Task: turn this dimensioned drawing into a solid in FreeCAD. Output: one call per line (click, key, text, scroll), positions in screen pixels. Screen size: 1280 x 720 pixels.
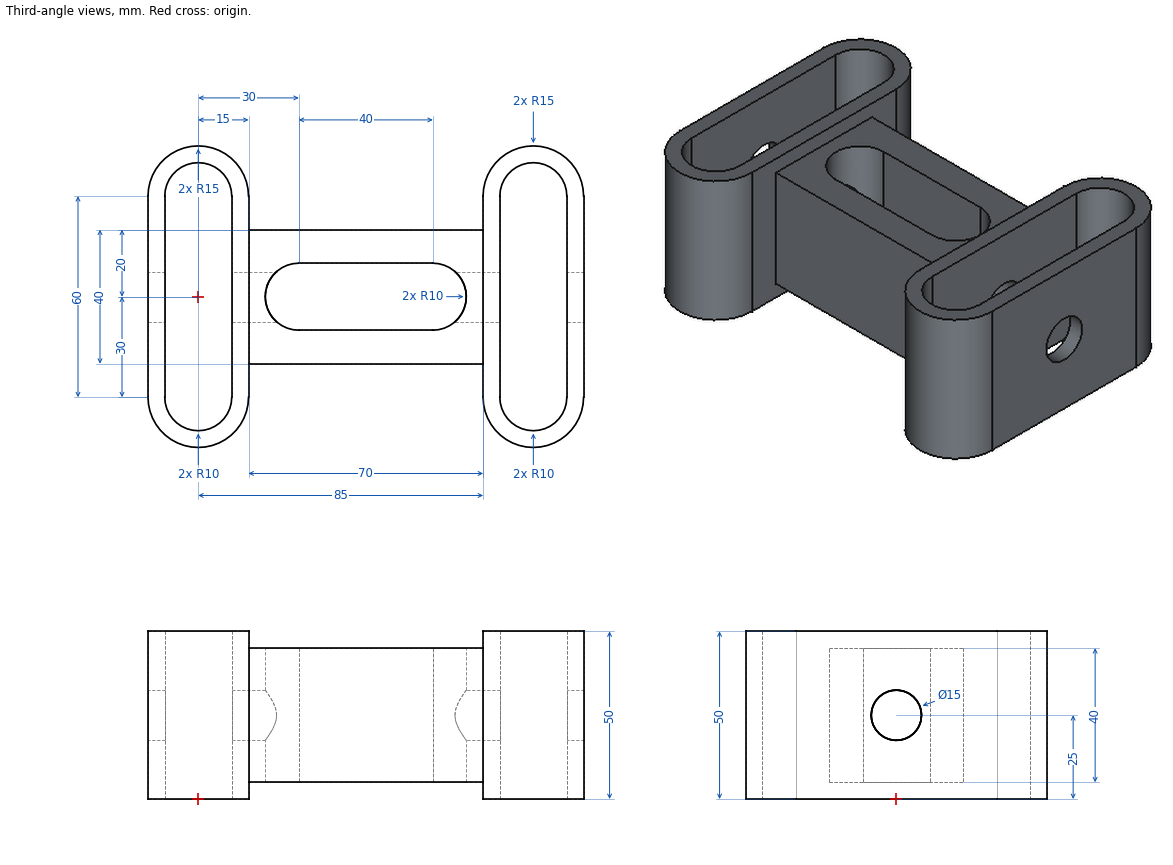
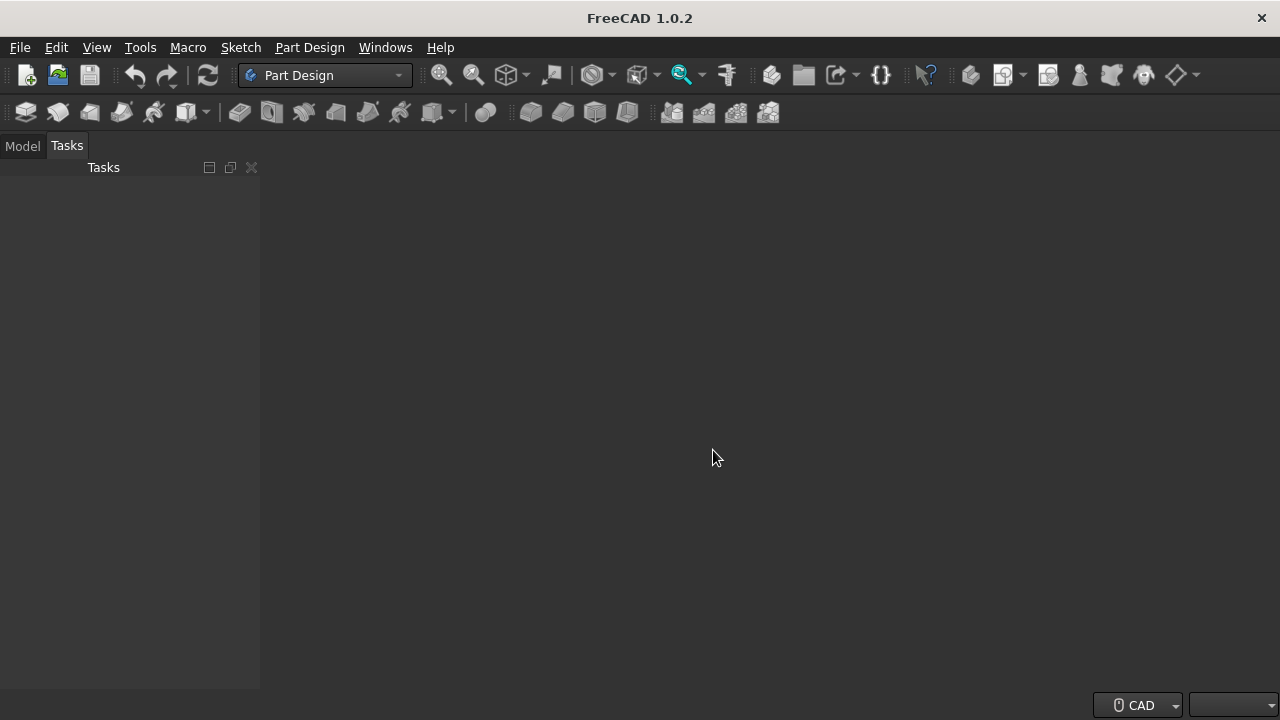
click(26, 76)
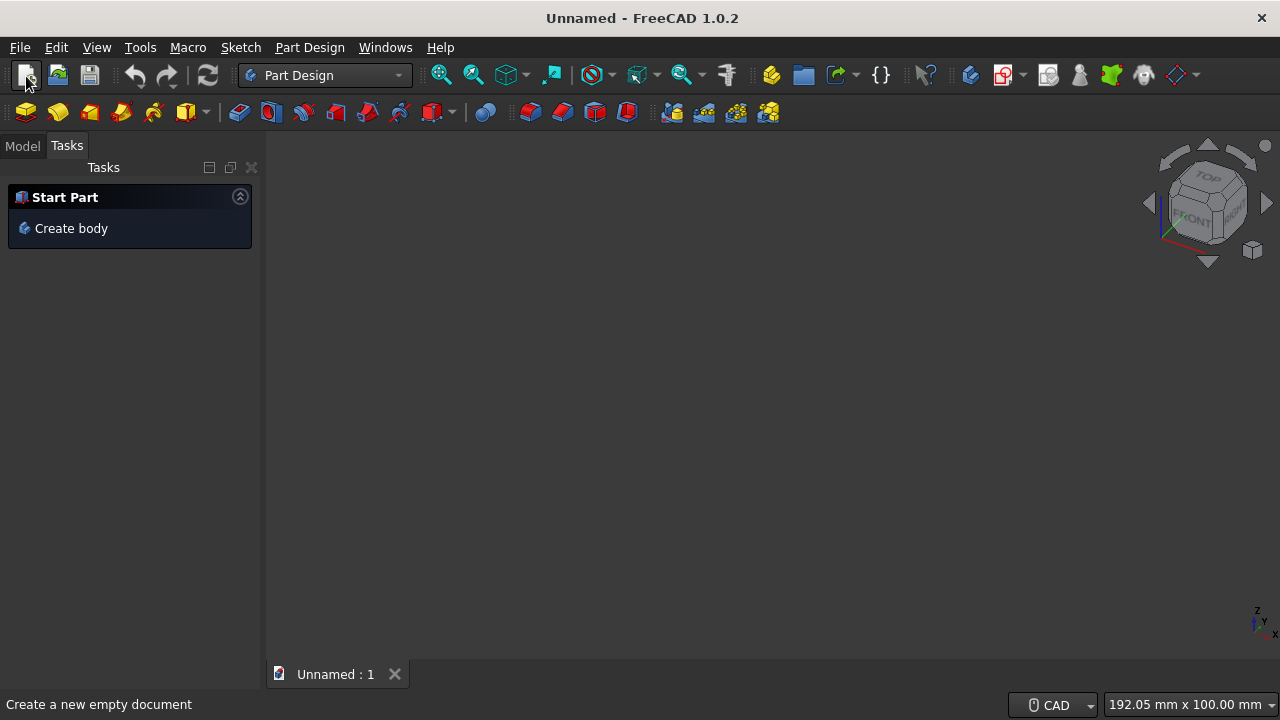
click(1004, 76)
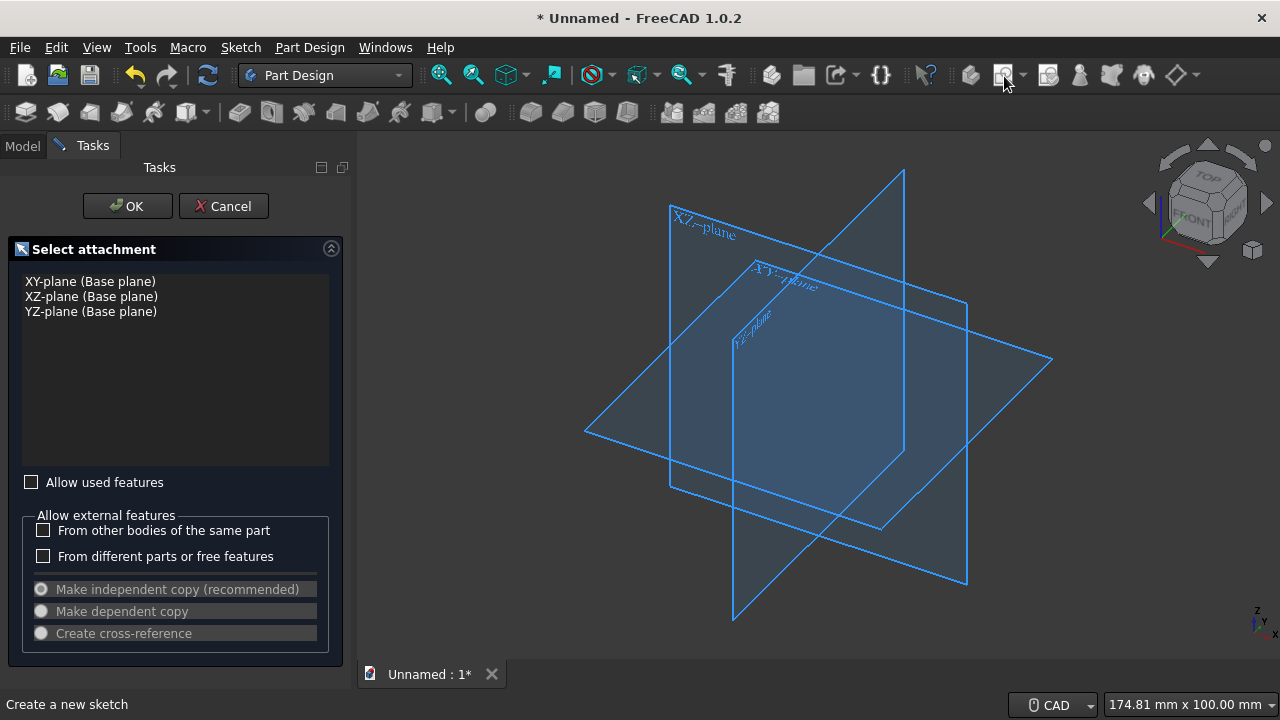
click(82, 282)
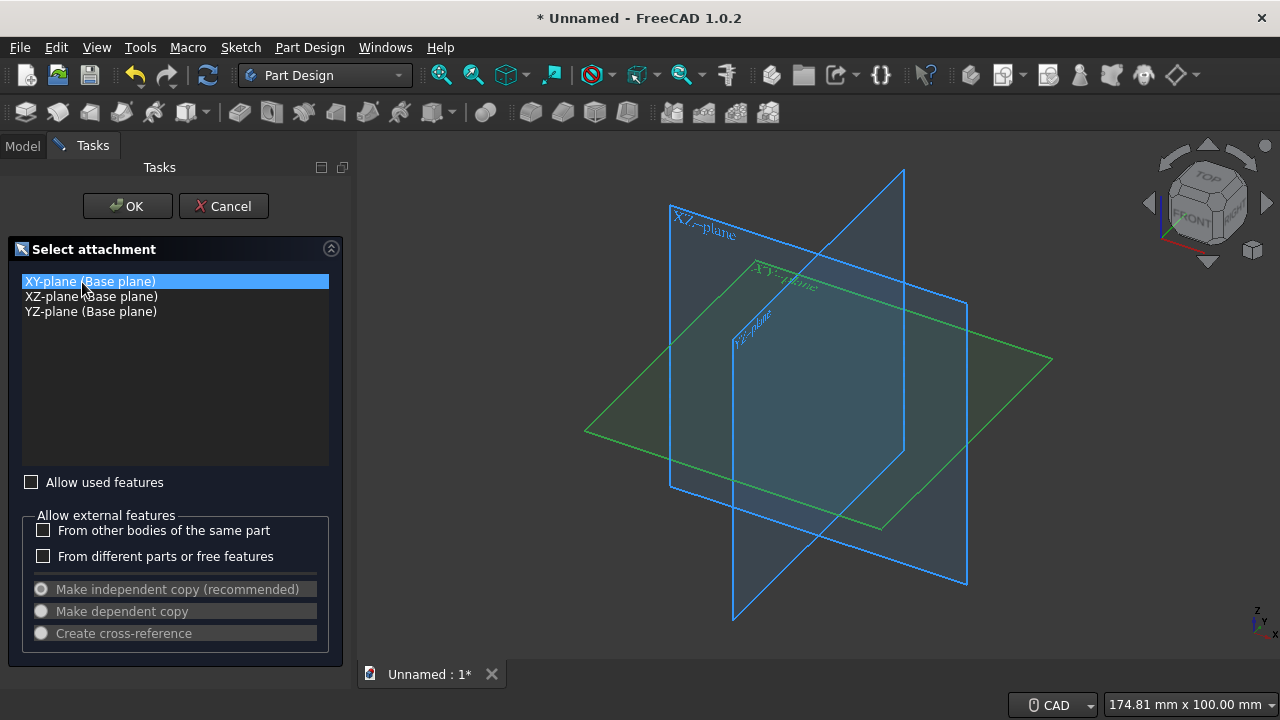
click(128, 206)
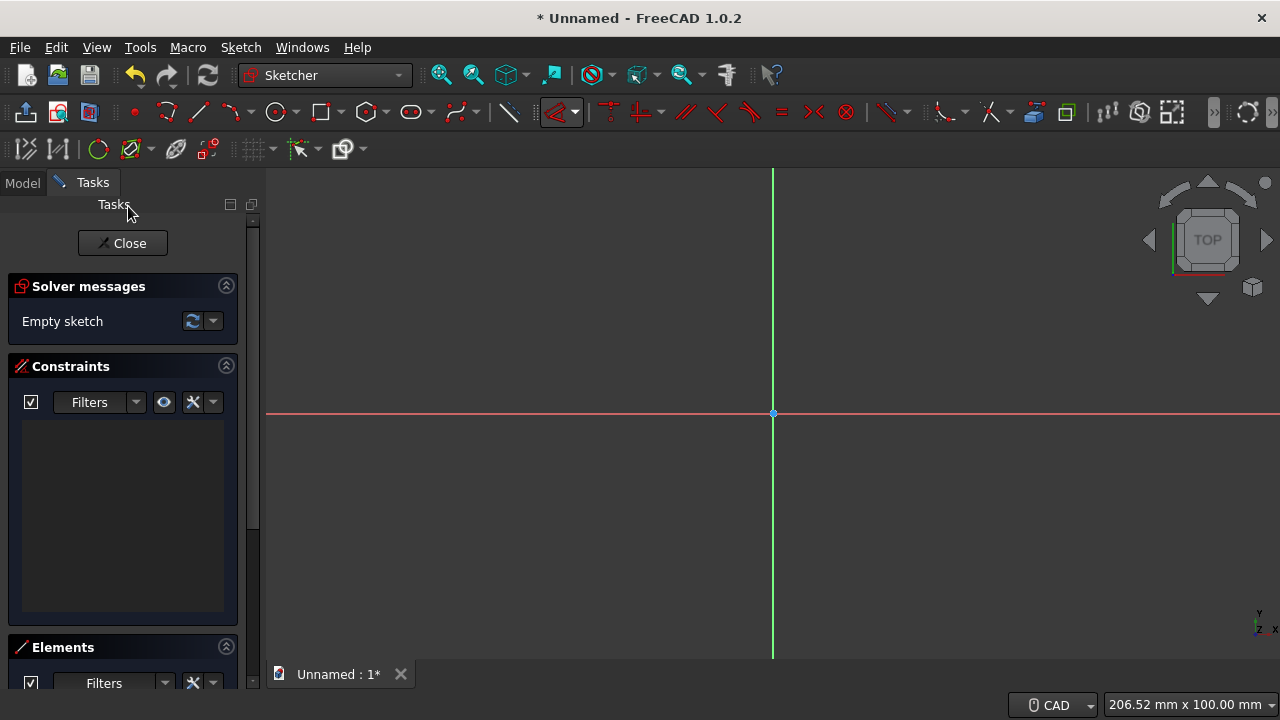
scroll(565, 414, down, 2)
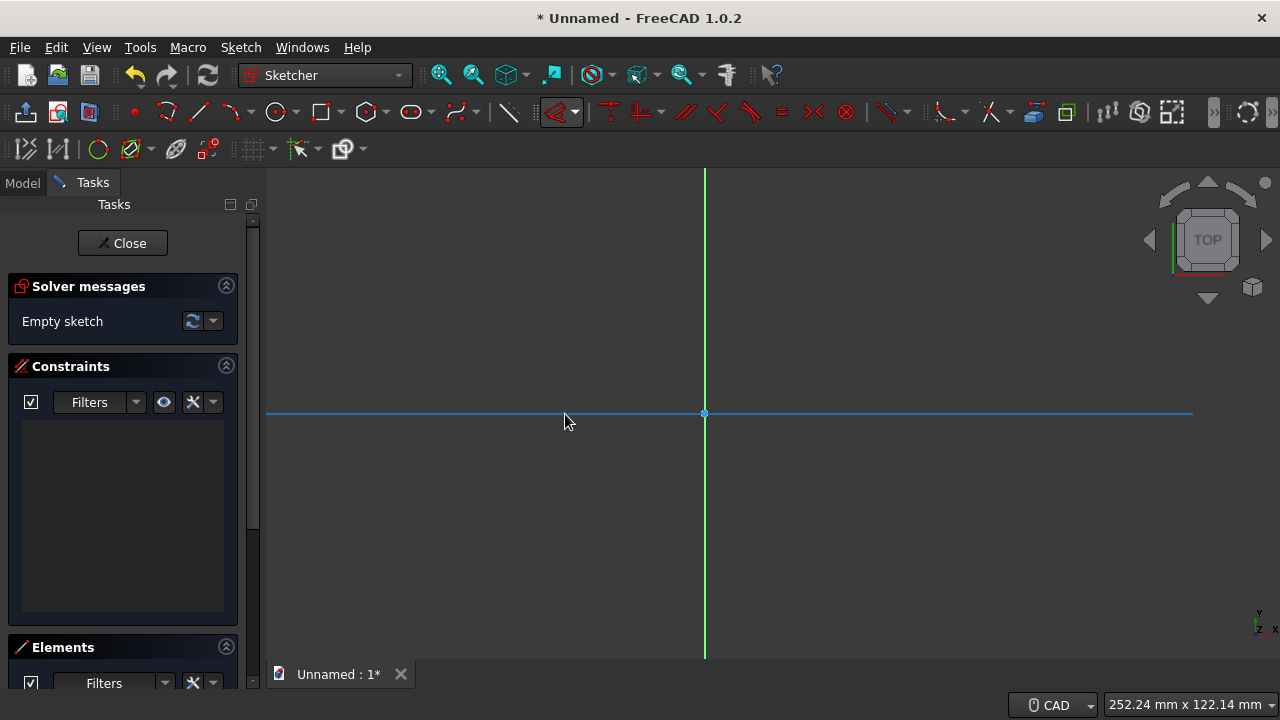
click(412, 112)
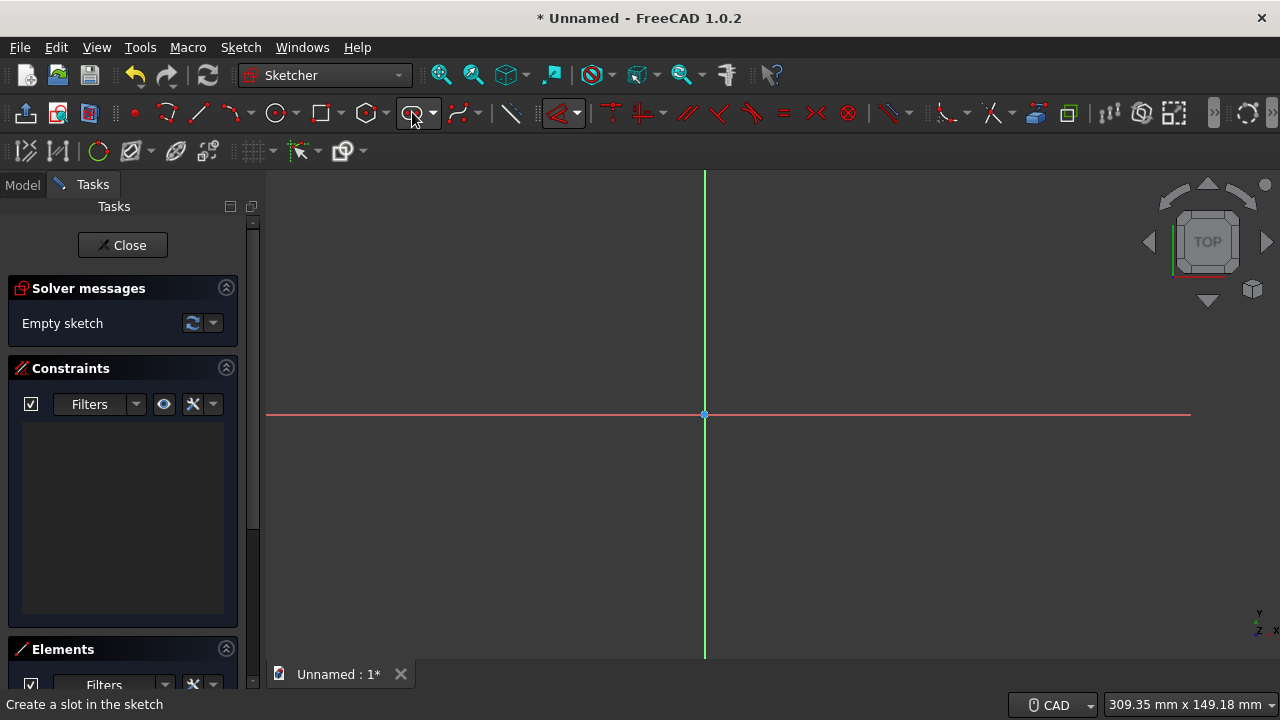
click(705, 513)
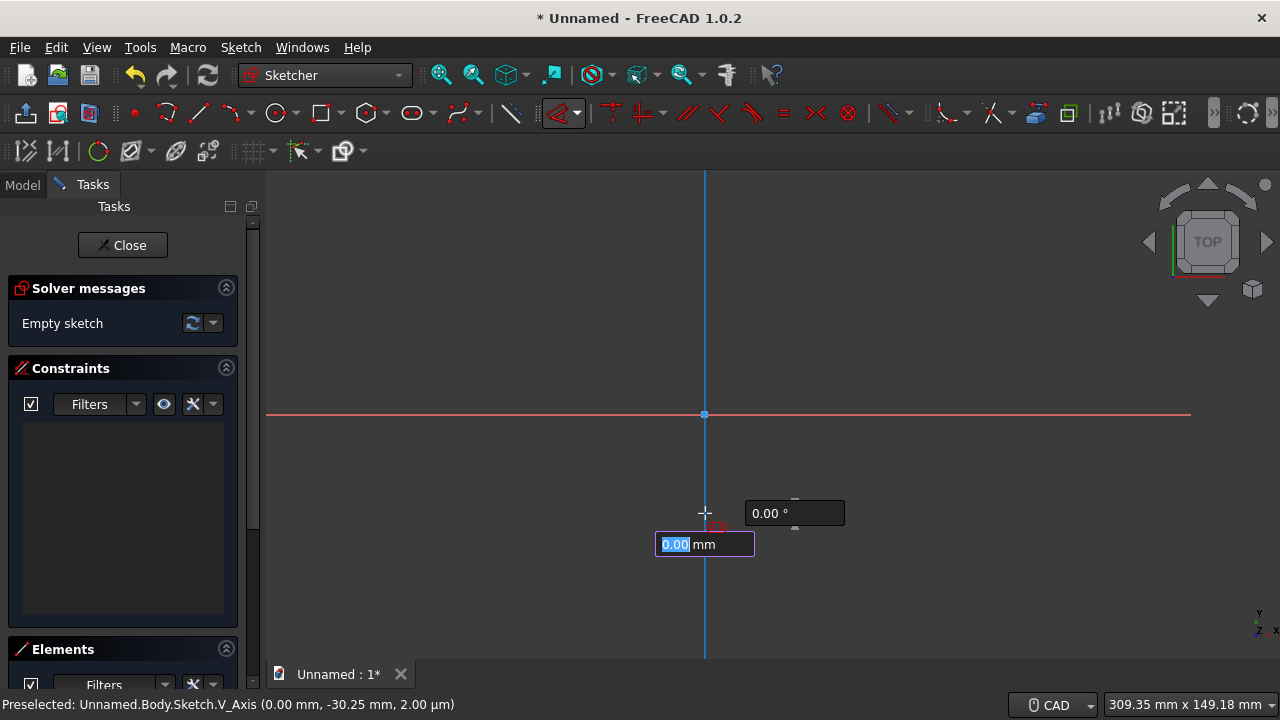
click(714, 316)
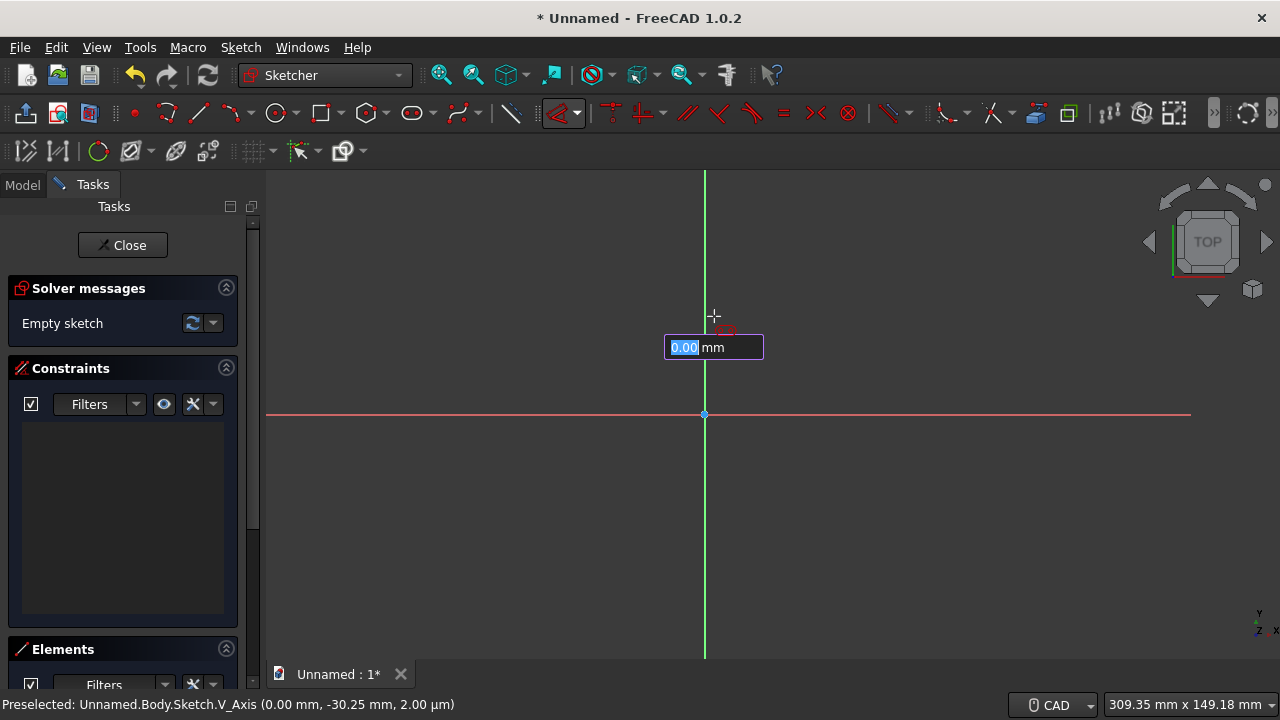
click(754, 444)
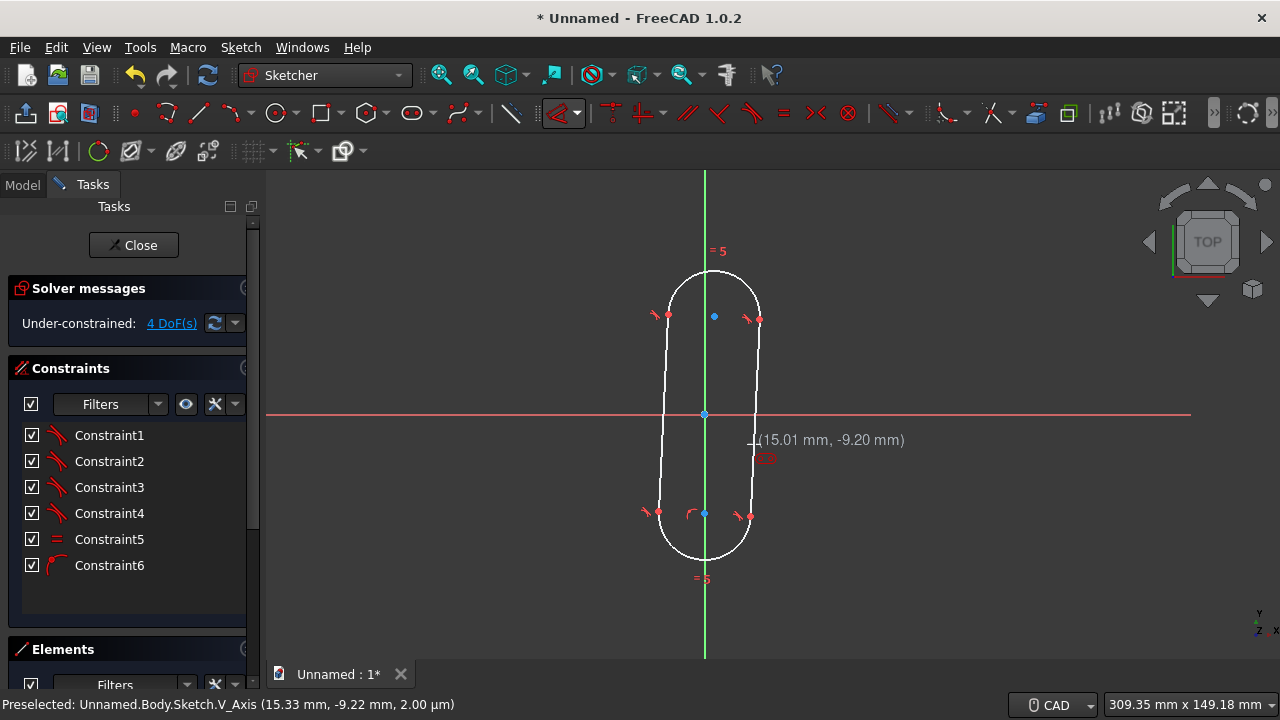
click(705, 514)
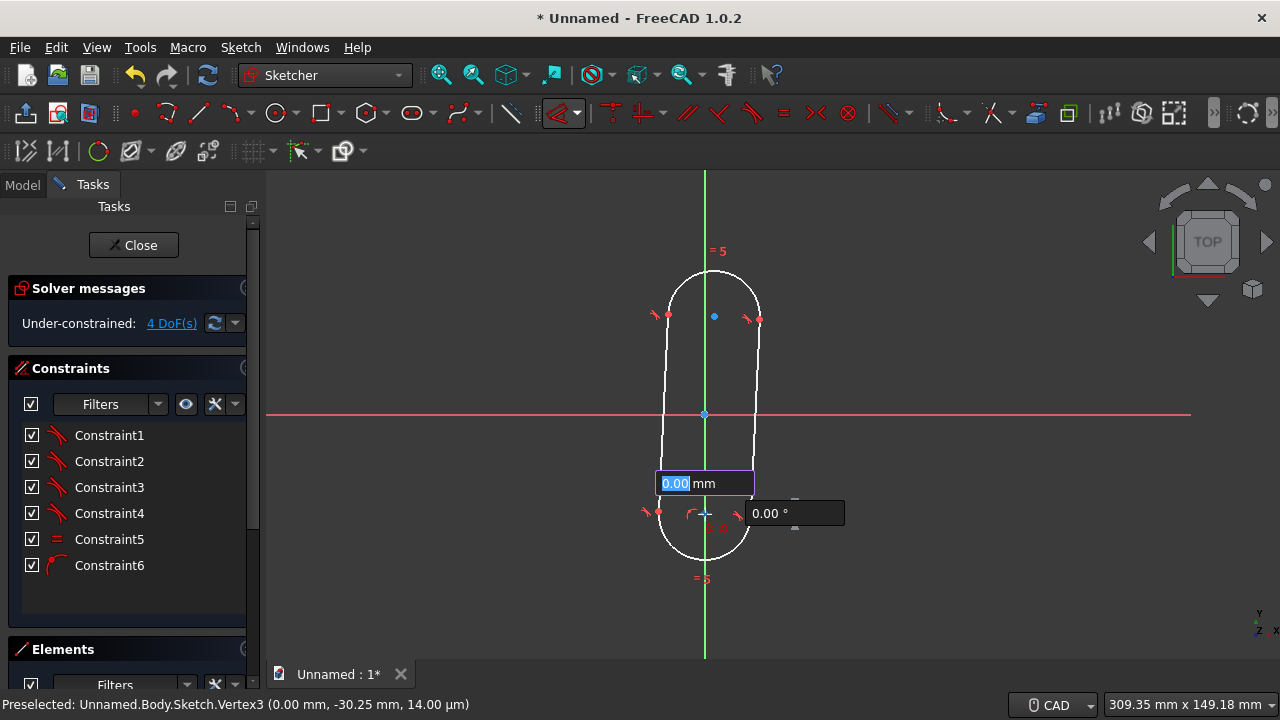
click(714, 317)